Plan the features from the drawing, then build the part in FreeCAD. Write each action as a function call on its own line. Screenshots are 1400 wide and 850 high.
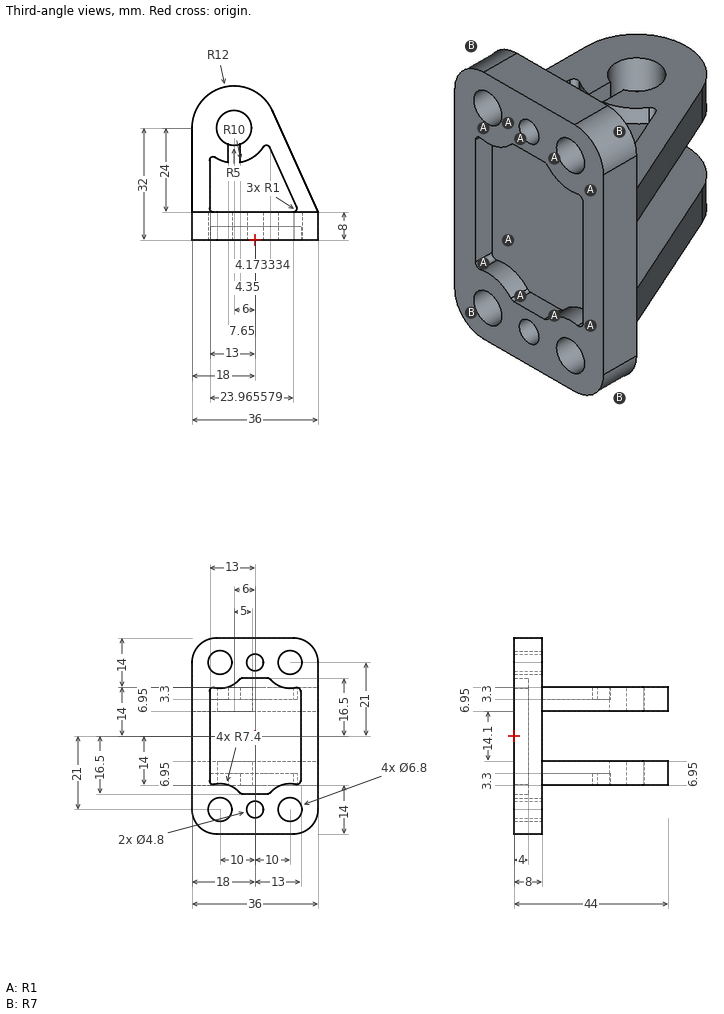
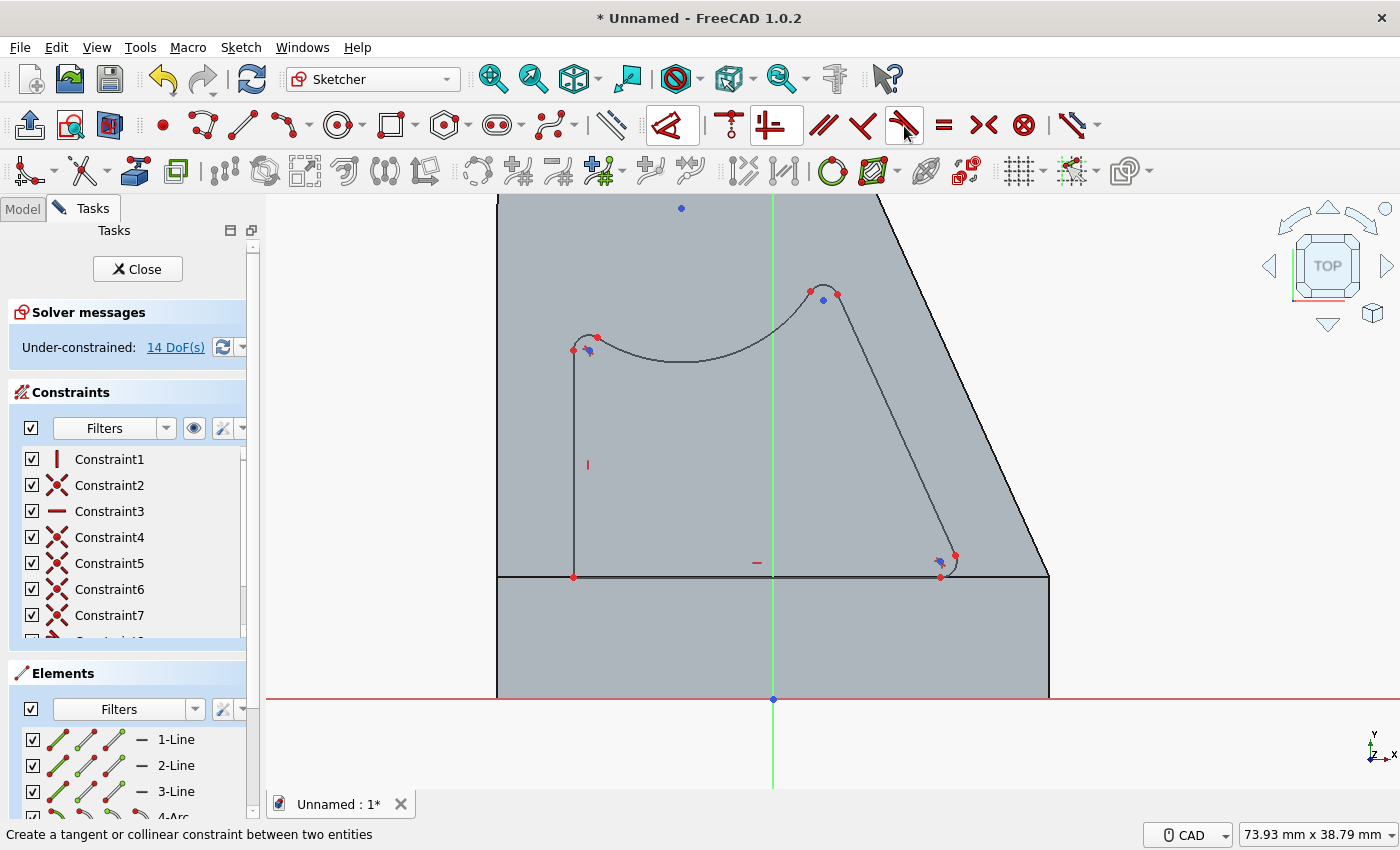
click(920, 477)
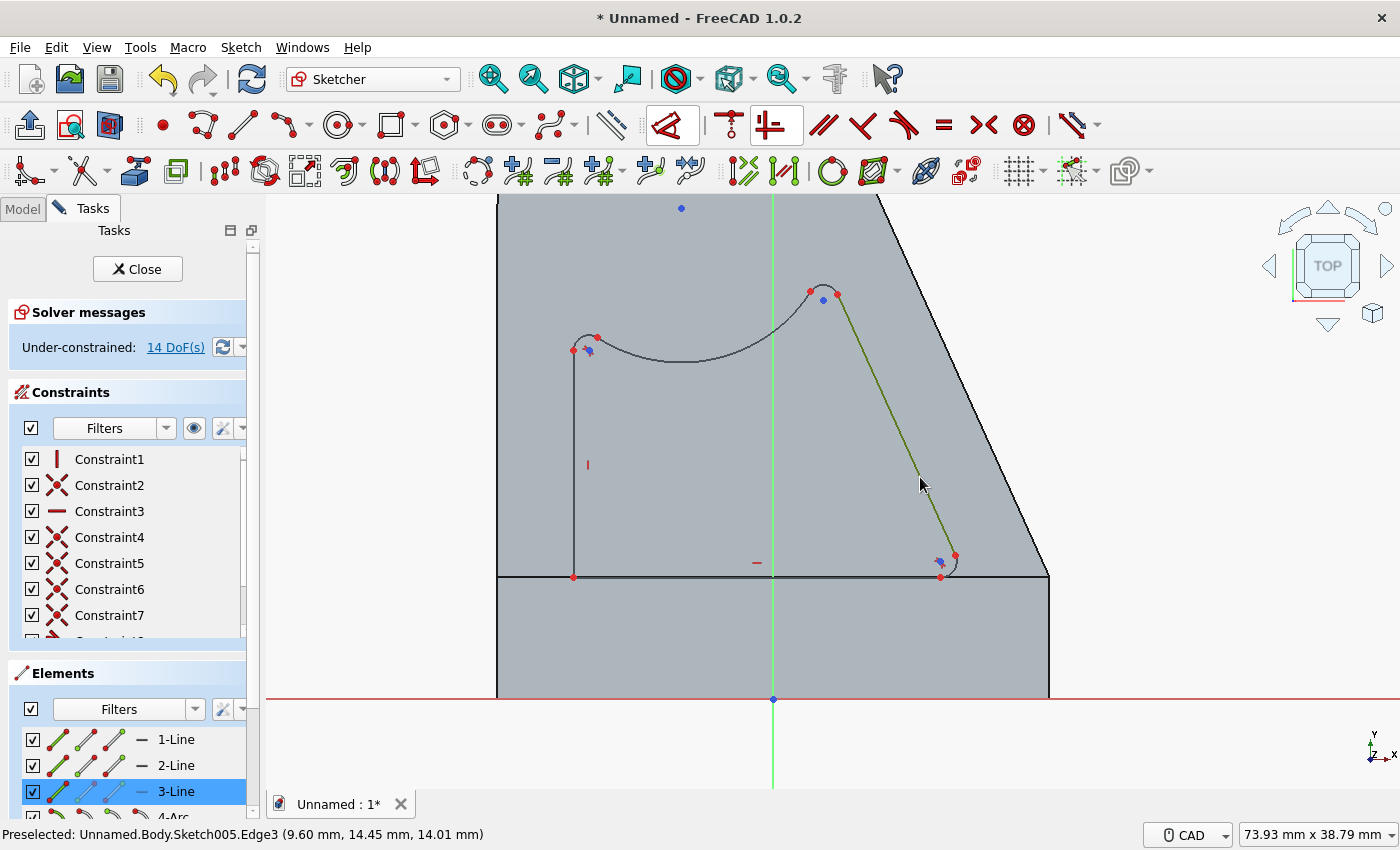
scroll(949, 575, up, 2)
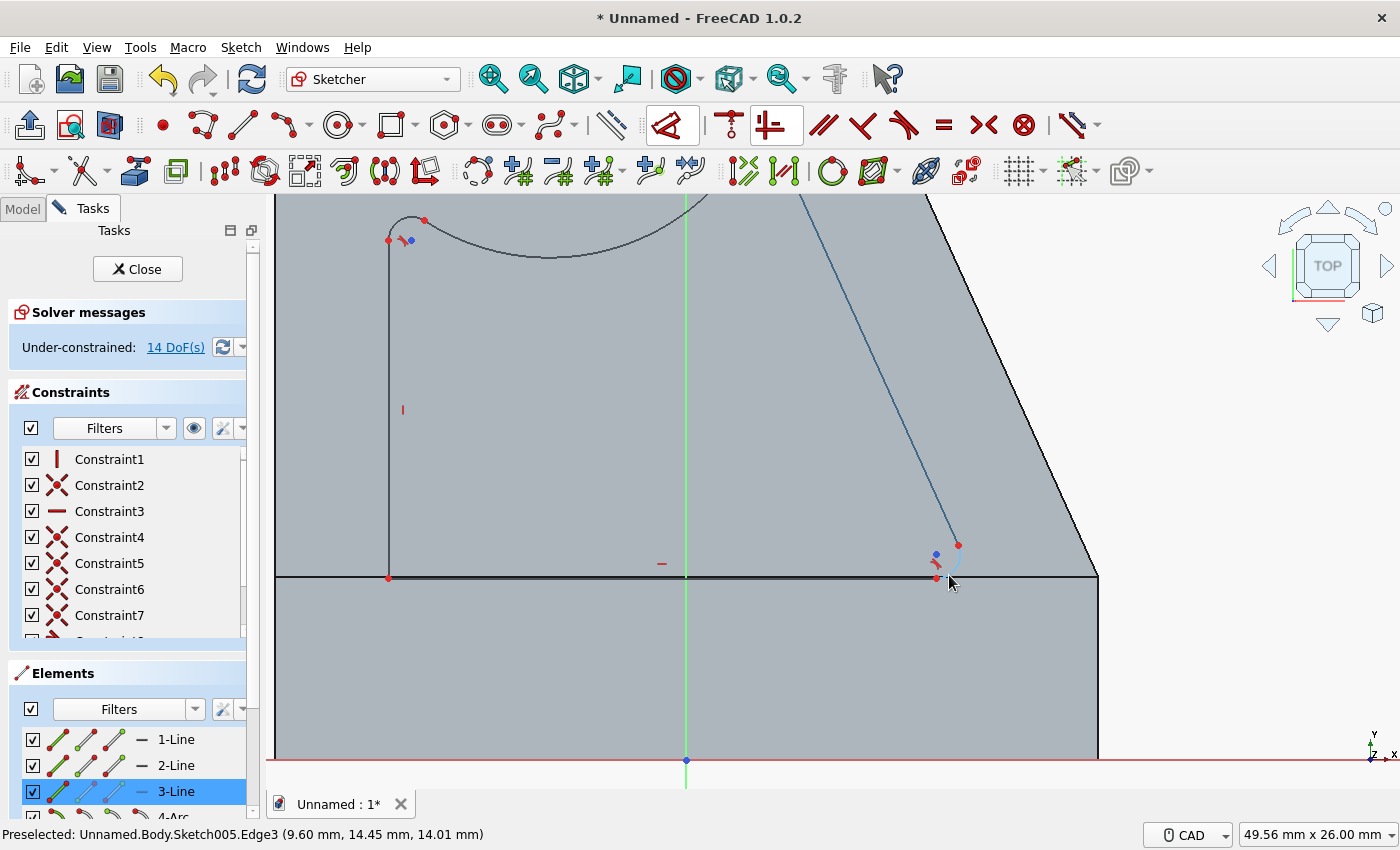
click(949, 575)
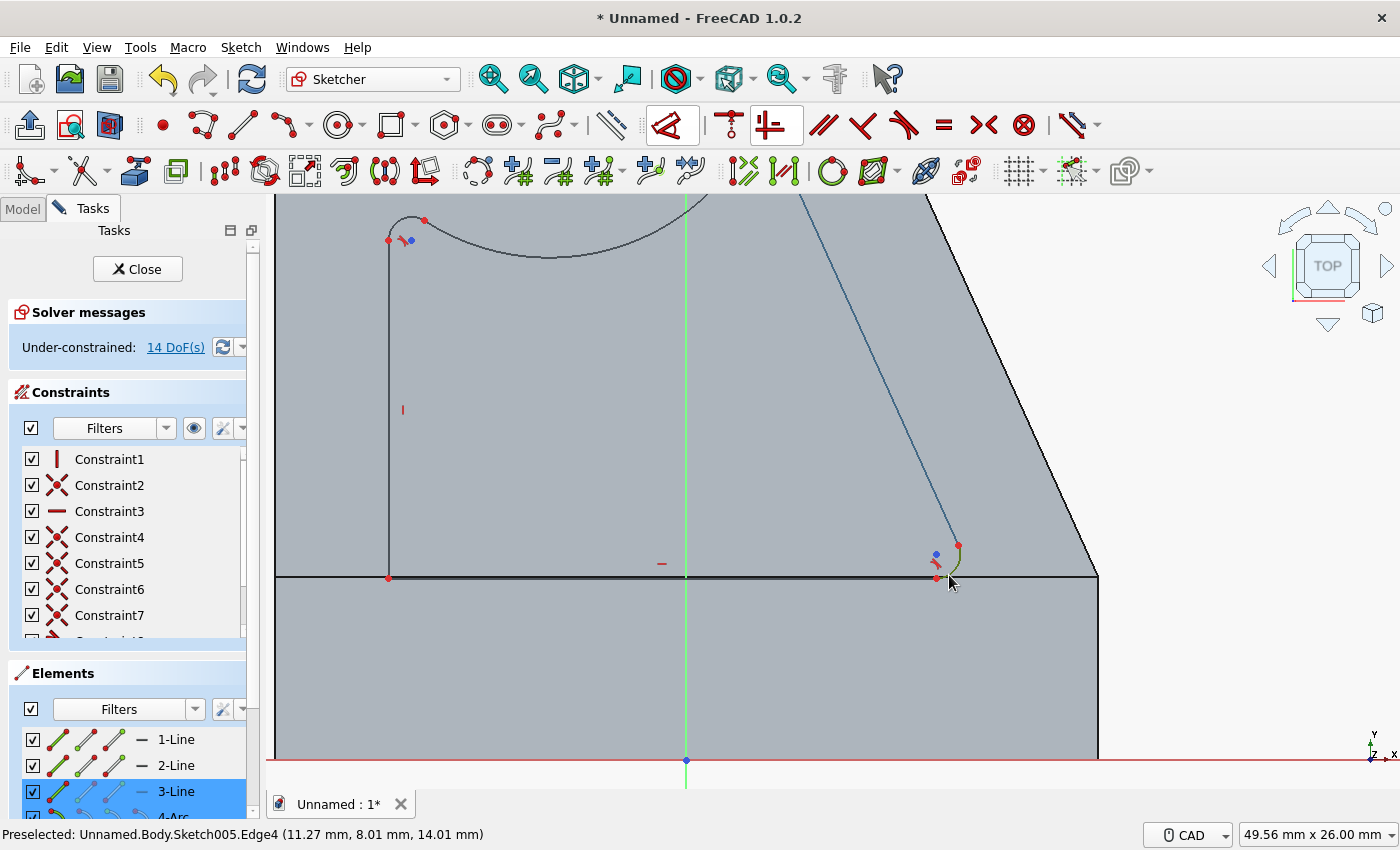
click(904, 126)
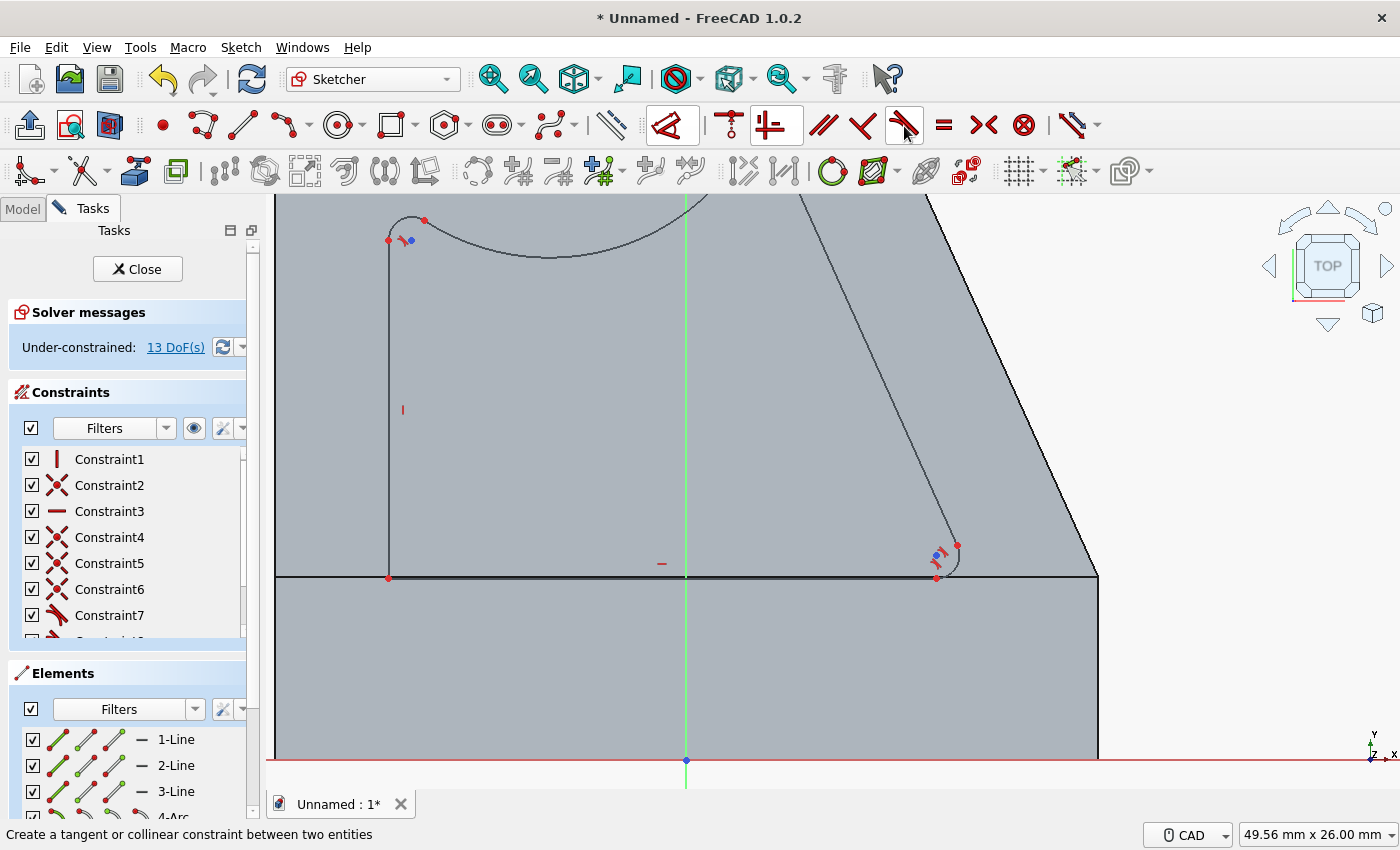
click(905, 429)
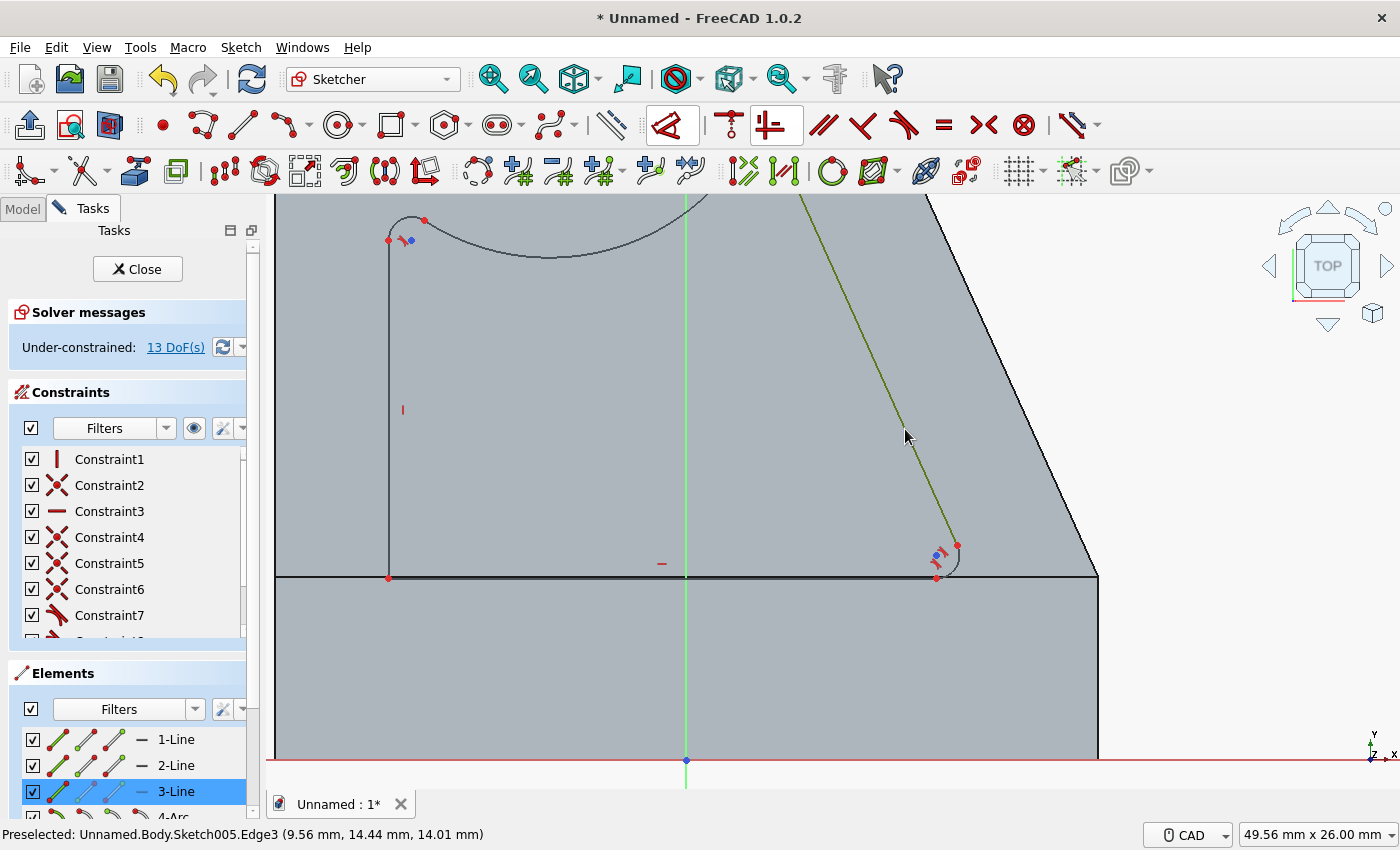
scroll(949, 574, down, 2)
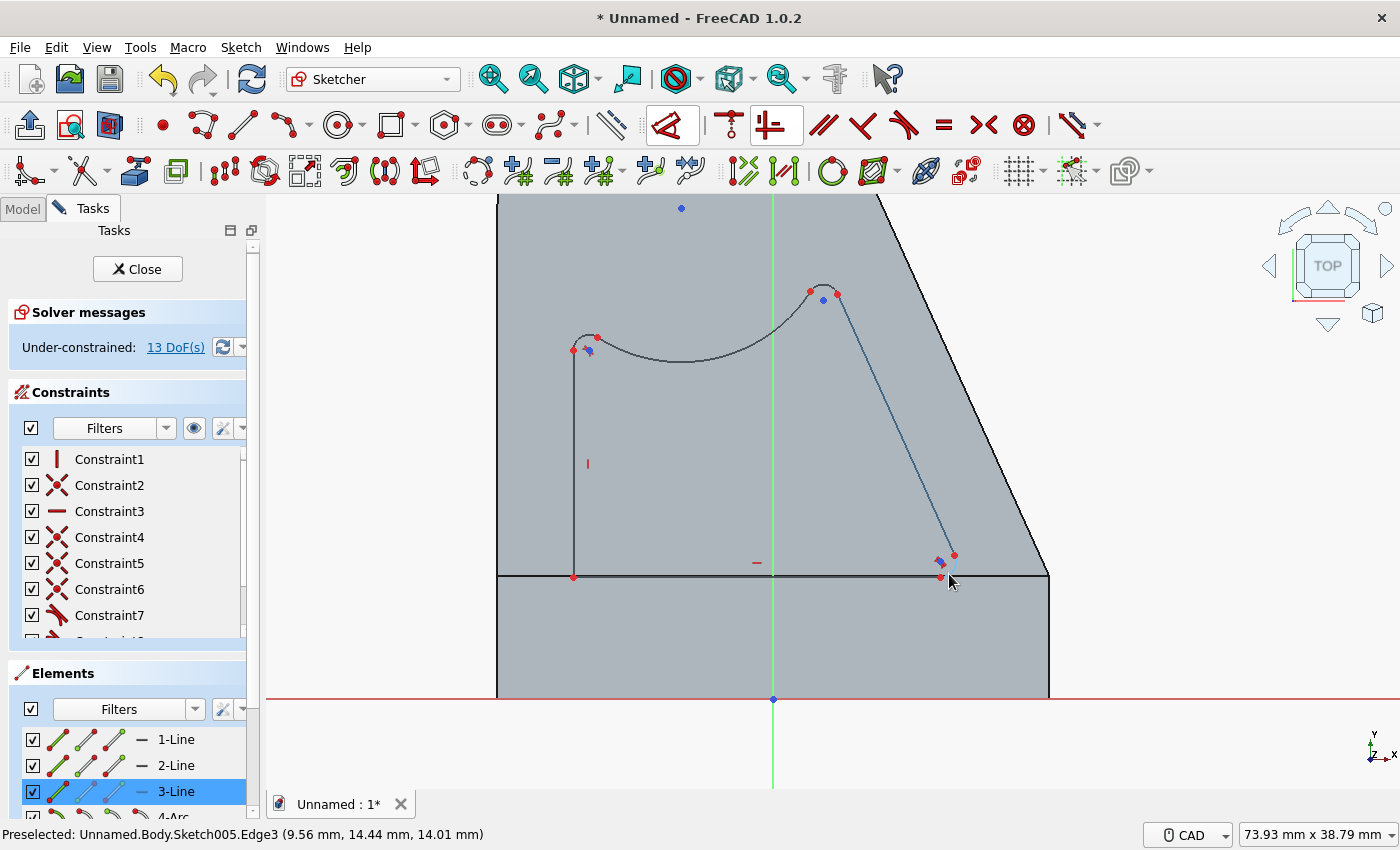
scroll(831, 287, up, 2)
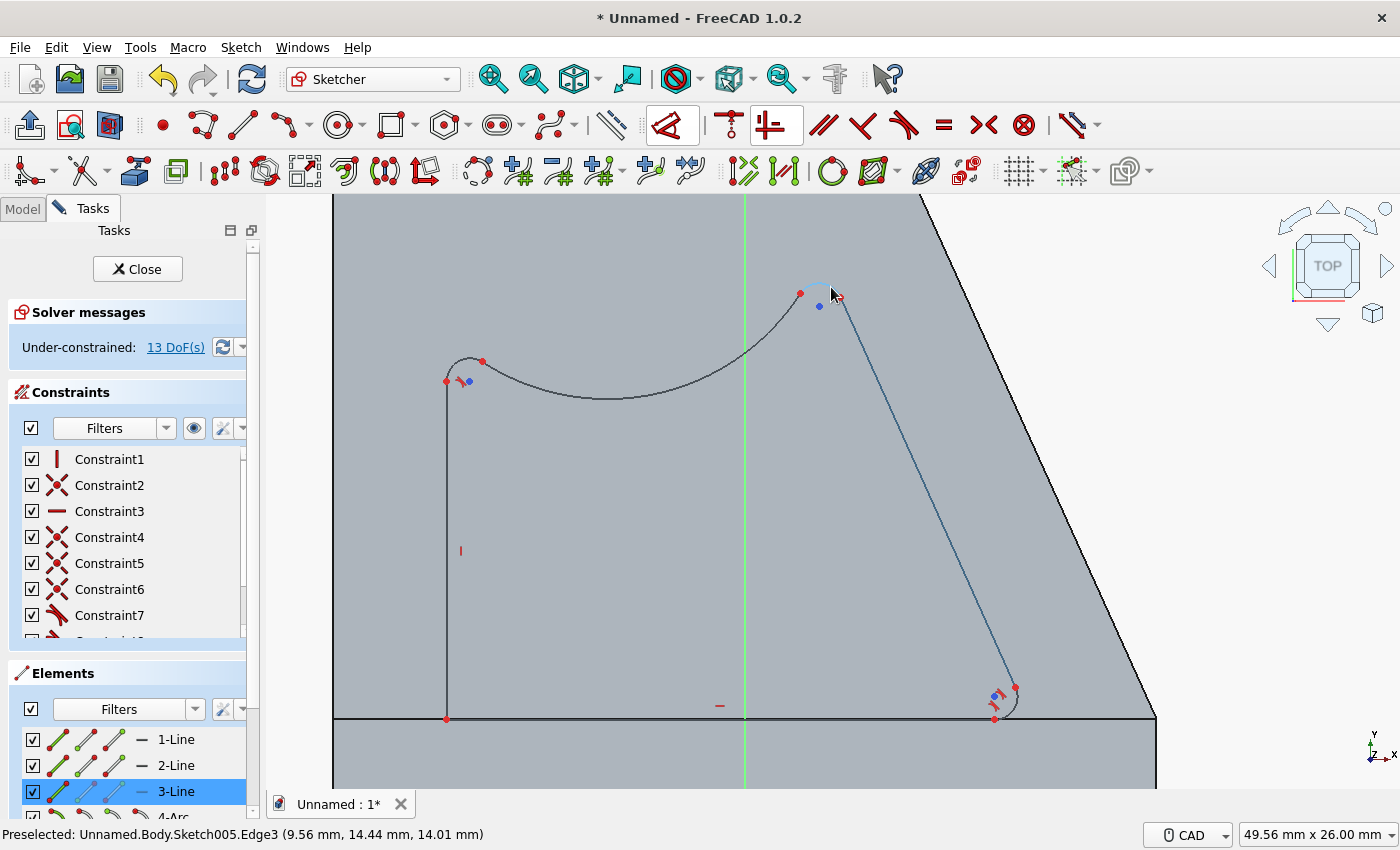
click(831, 287)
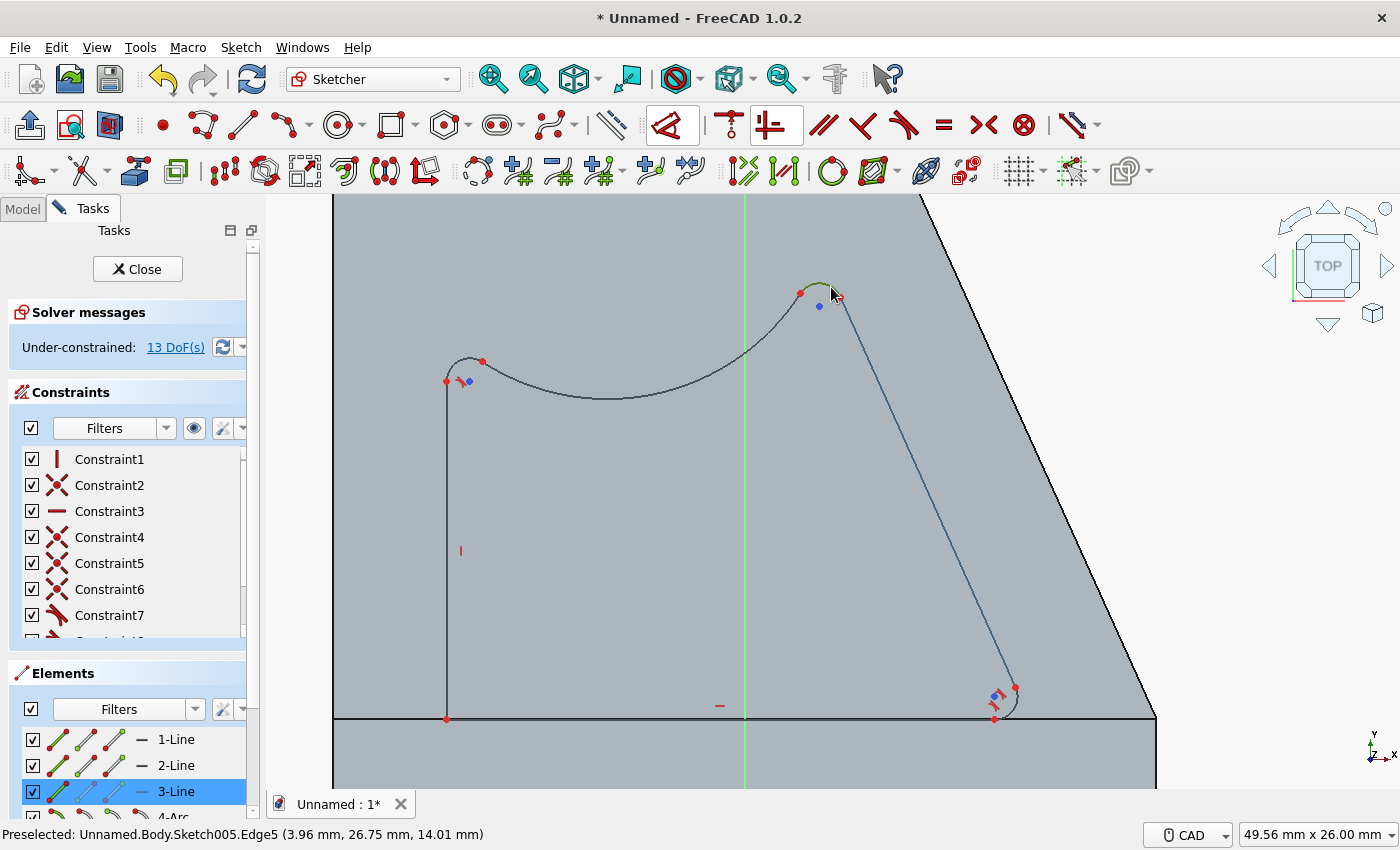
key(t)